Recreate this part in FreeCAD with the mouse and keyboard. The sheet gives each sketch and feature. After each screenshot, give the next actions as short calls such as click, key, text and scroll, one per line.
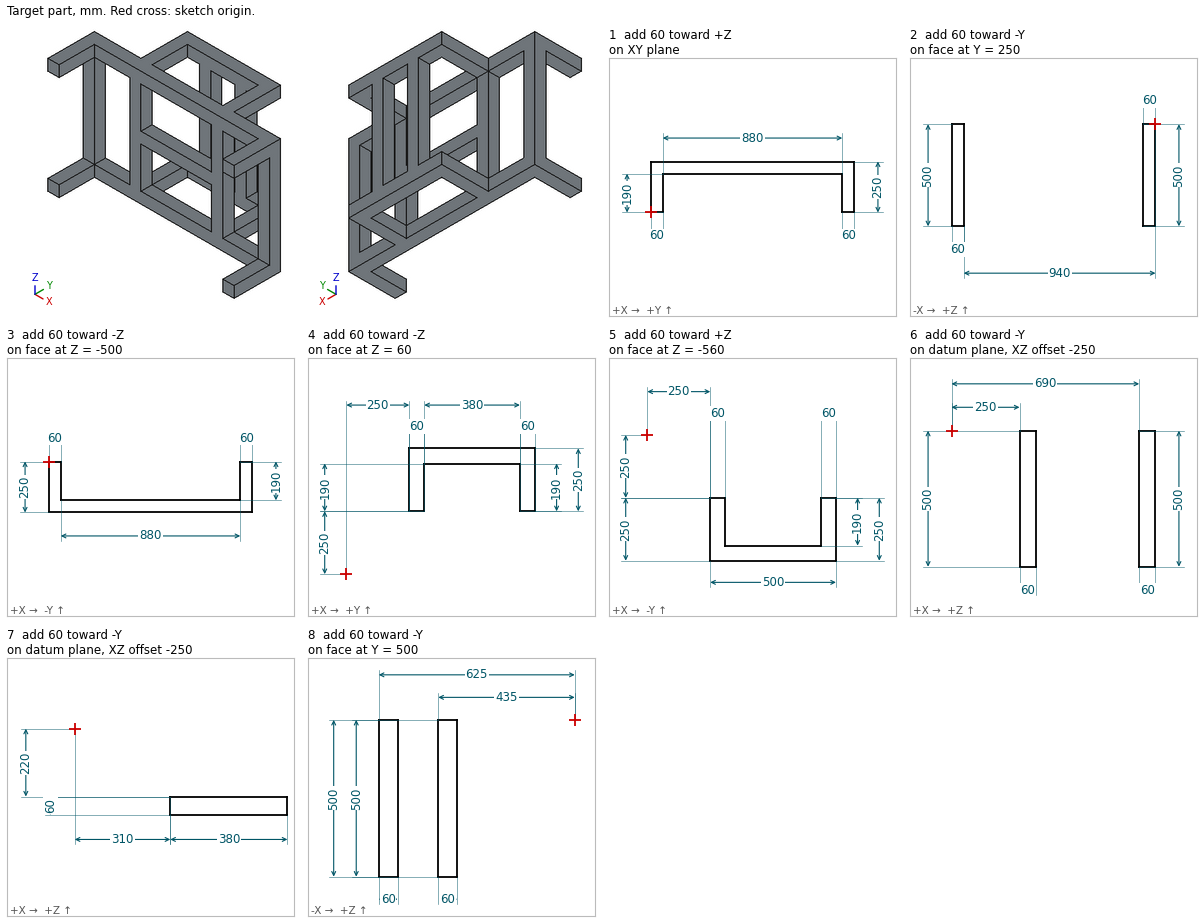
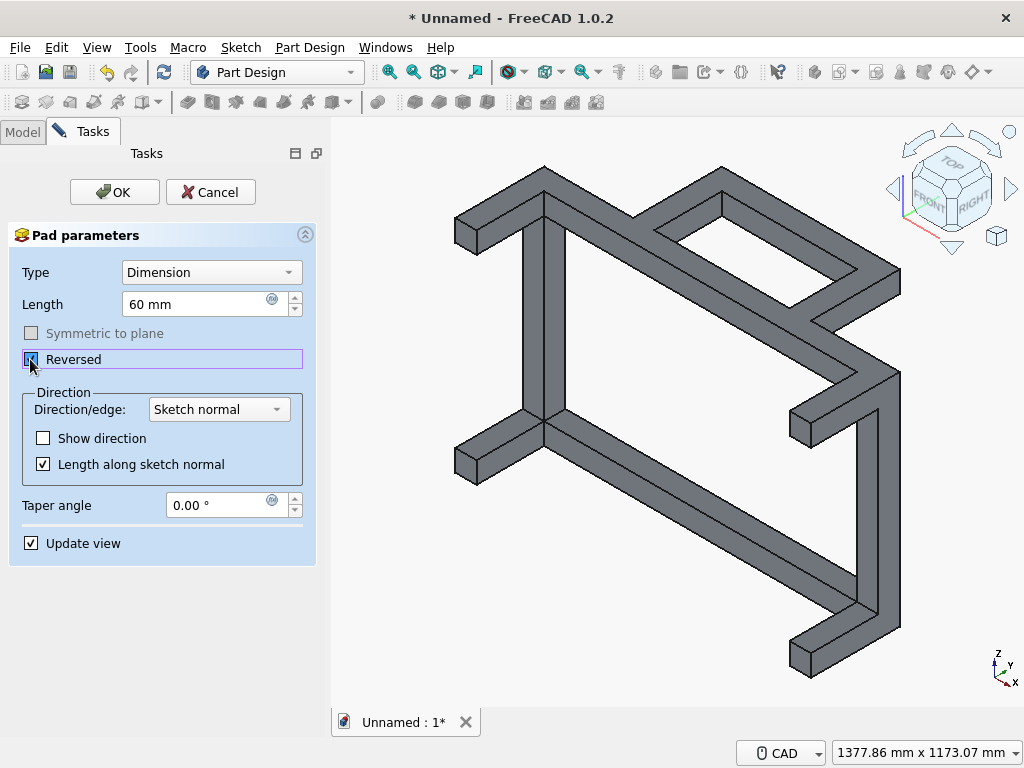
click(115, 192)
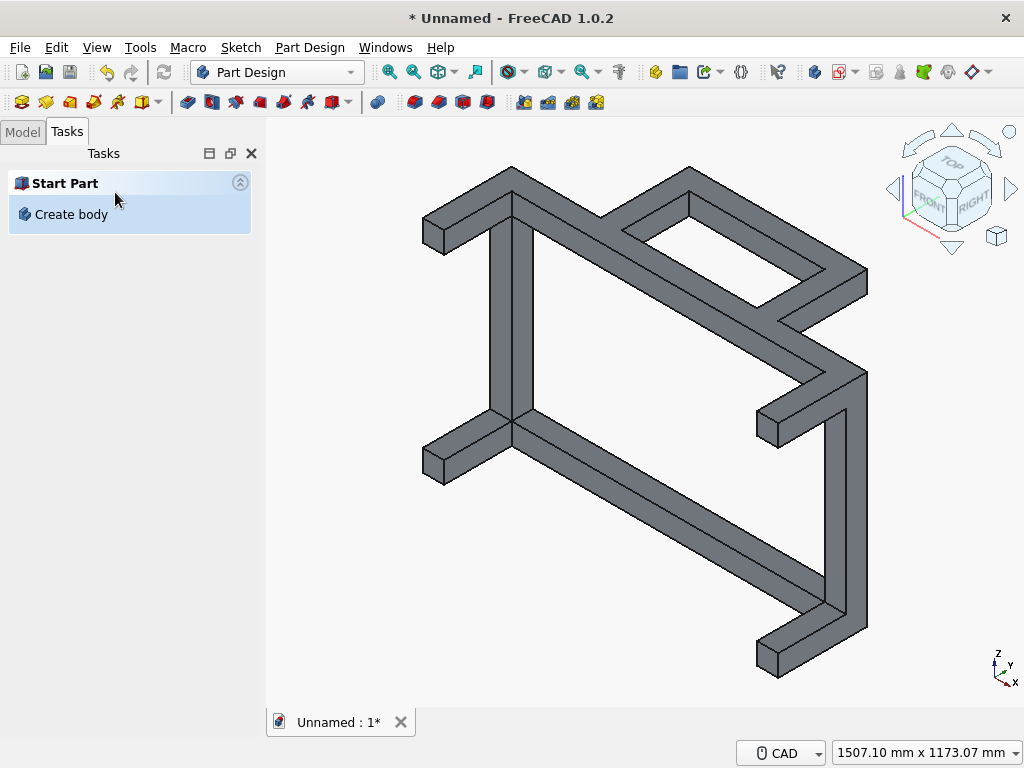
click(390, 72)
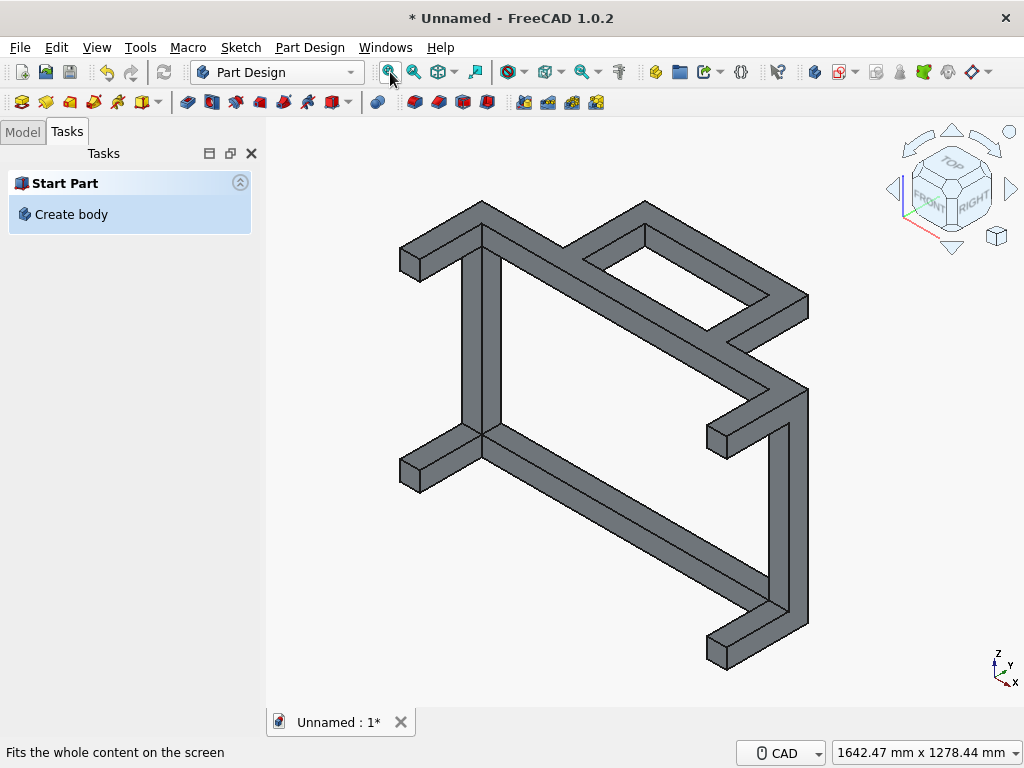
key(5)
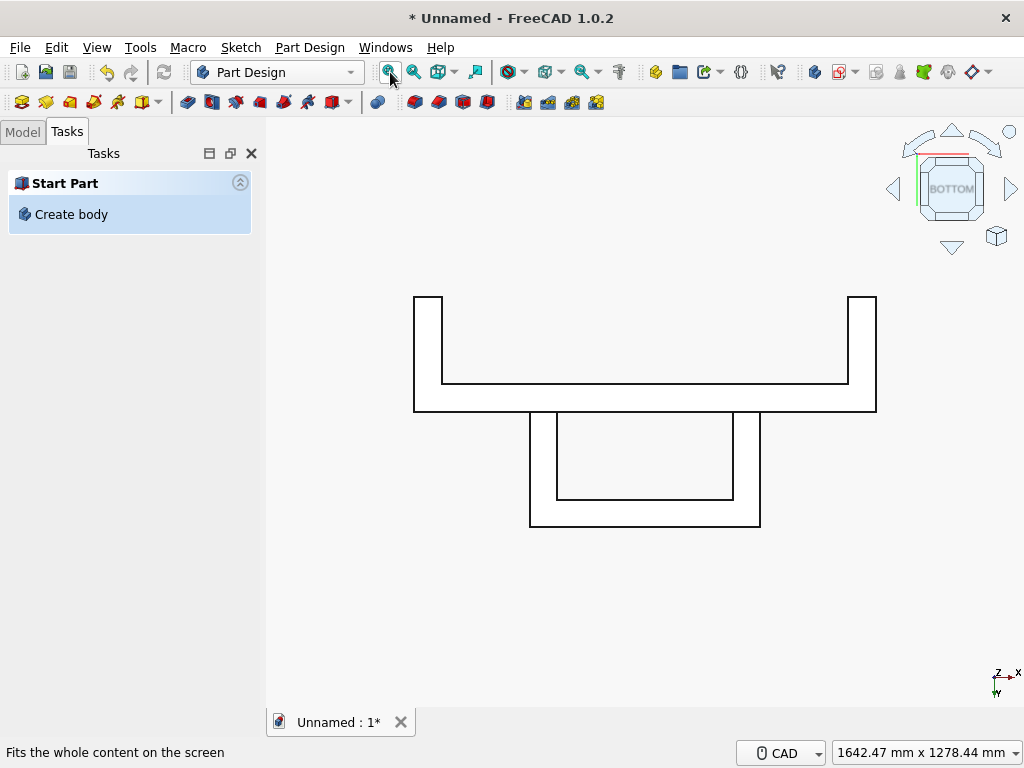
click(843, 403)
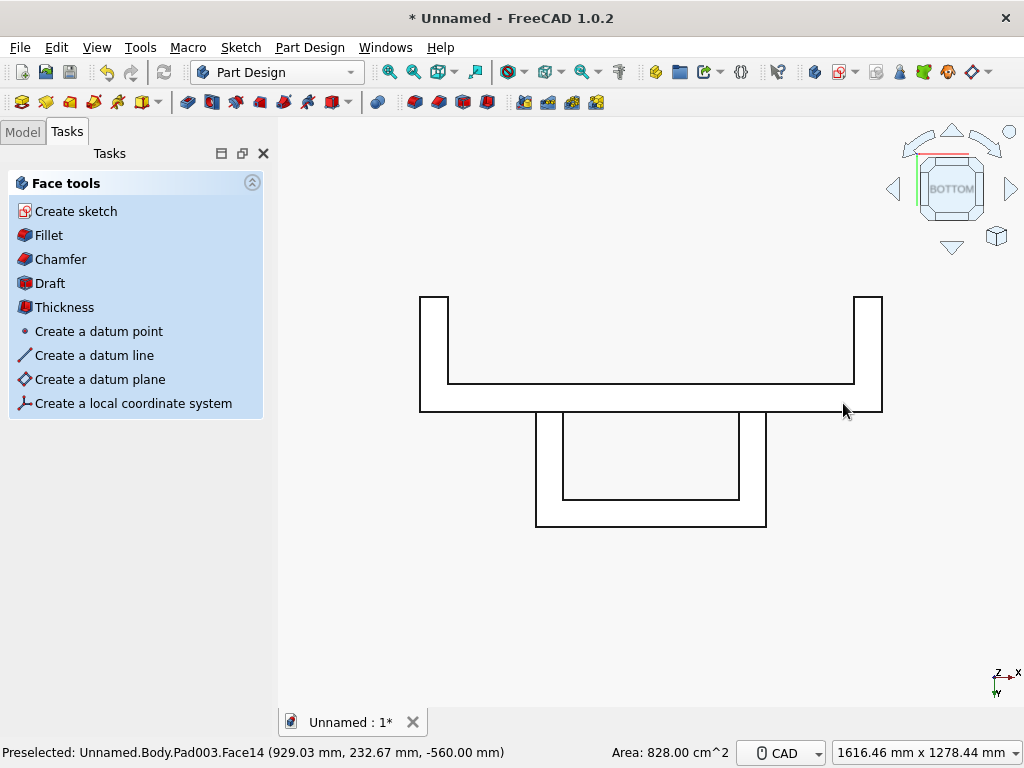
click(840, 72)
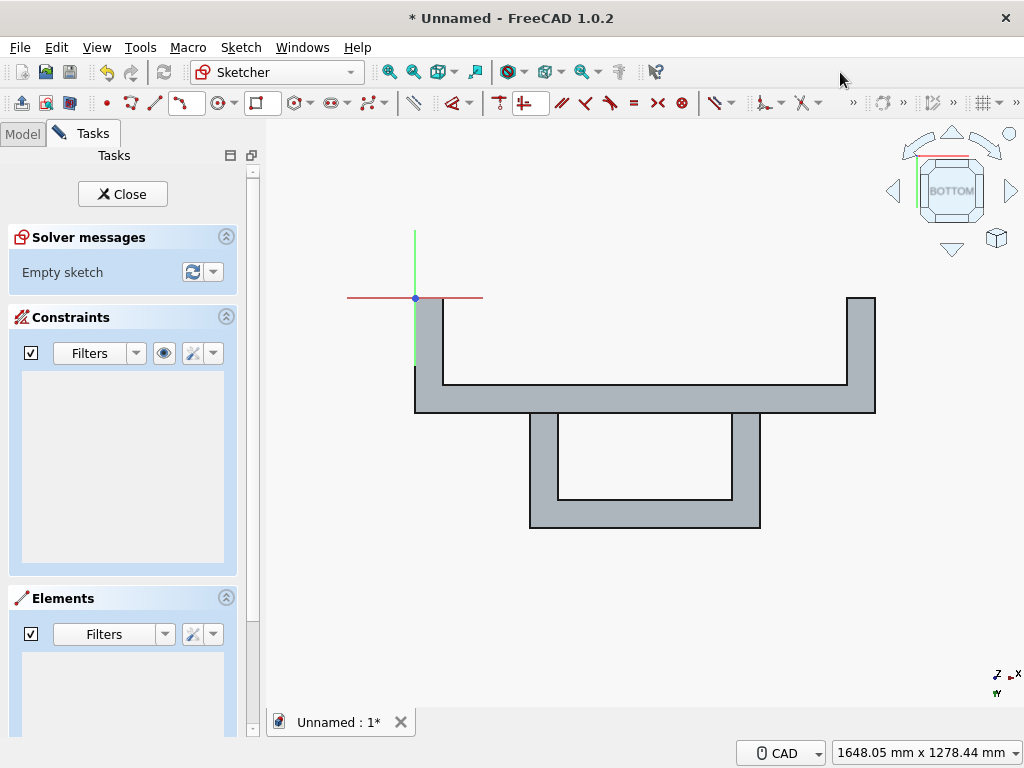
click(132, 104)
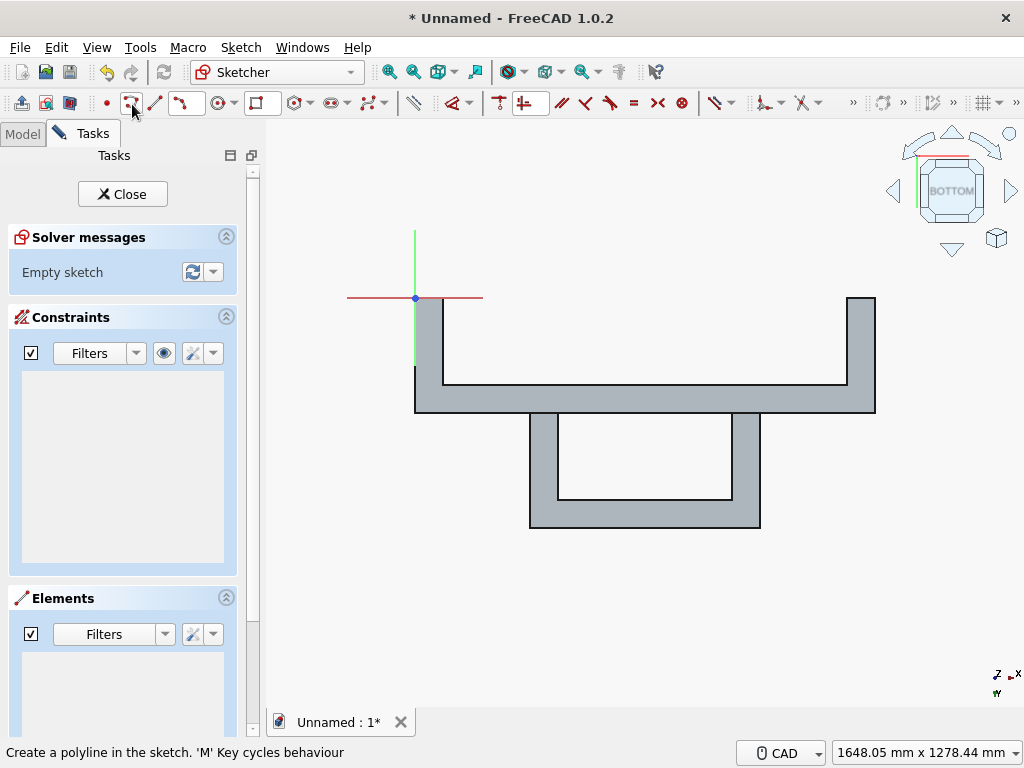
click(530, 413)
click(530, 528)
click(760, 528)
click(760, 413)
click(732, 413)
click(732, 500)
click(558, 500)
click(558, 413)
click(530, 414)
key(Escape)
key(Escape)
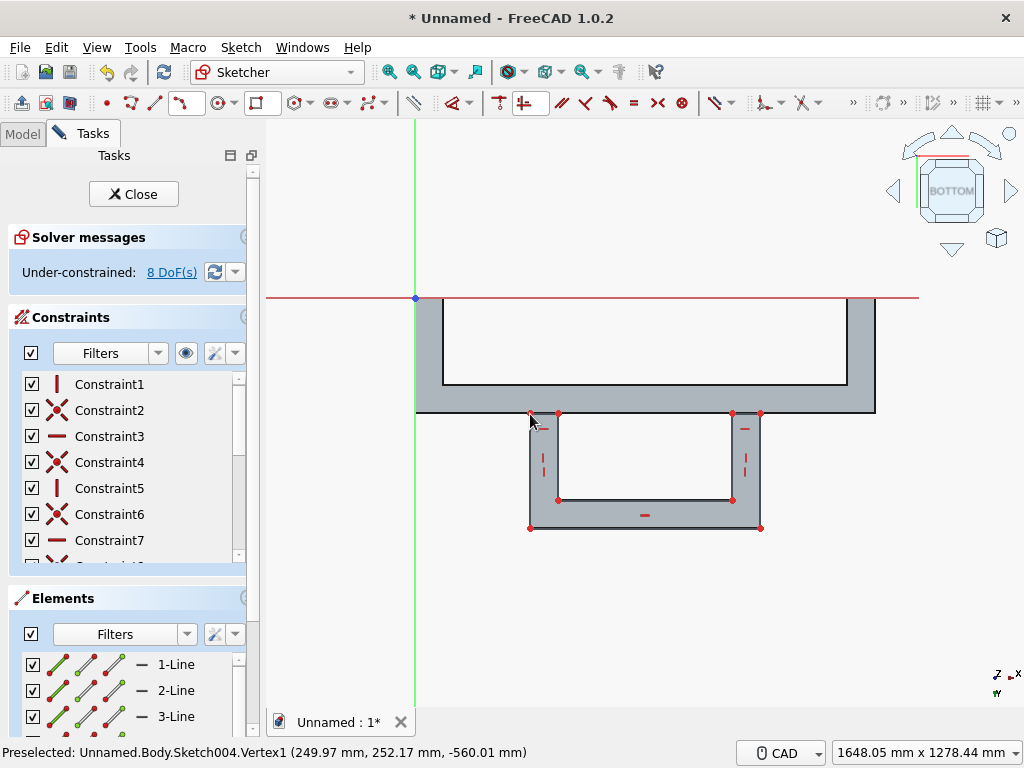
click(452, 104)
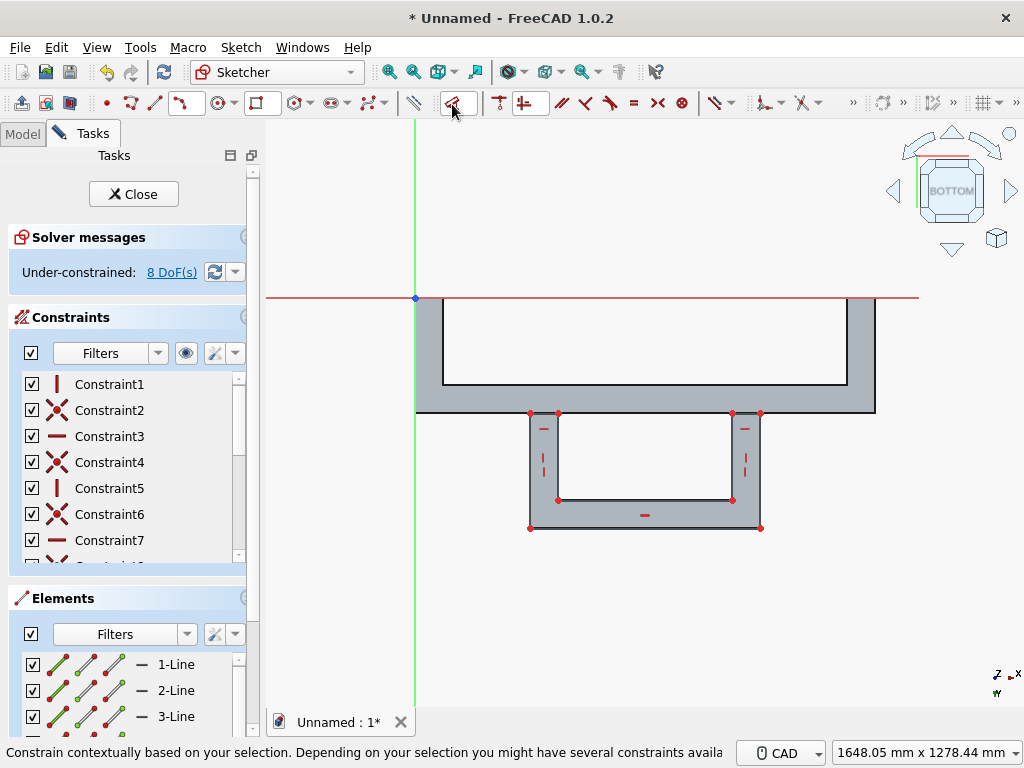
scroll(749, 414, up, 2)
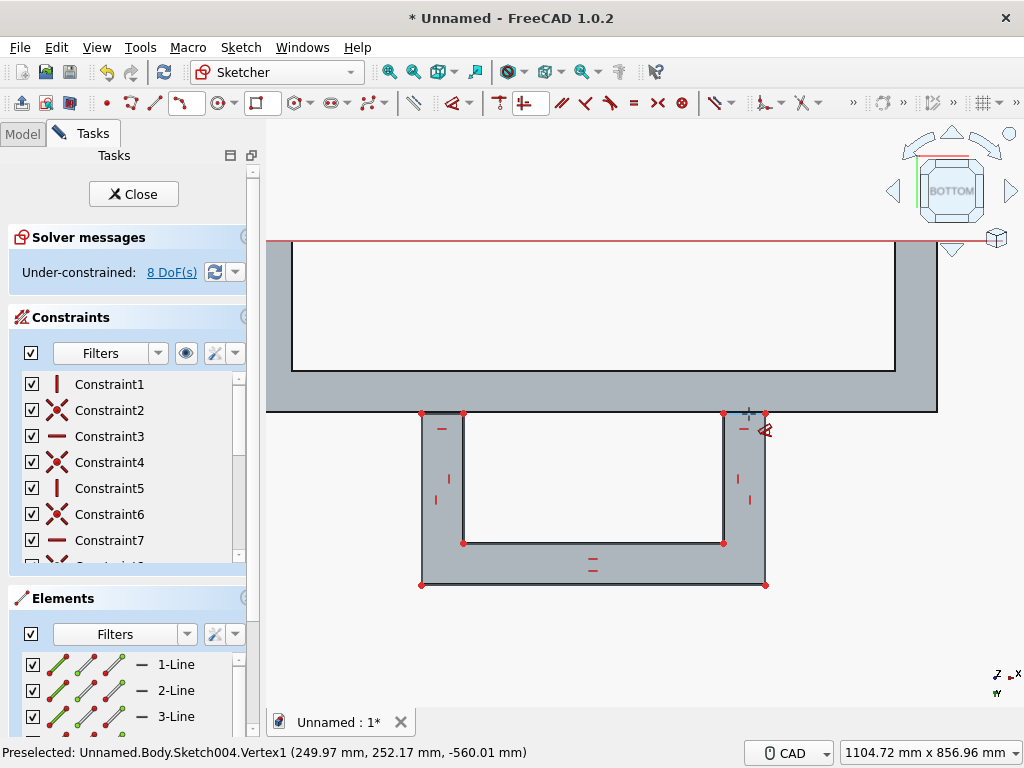
click(748, 414)
click(744, 448)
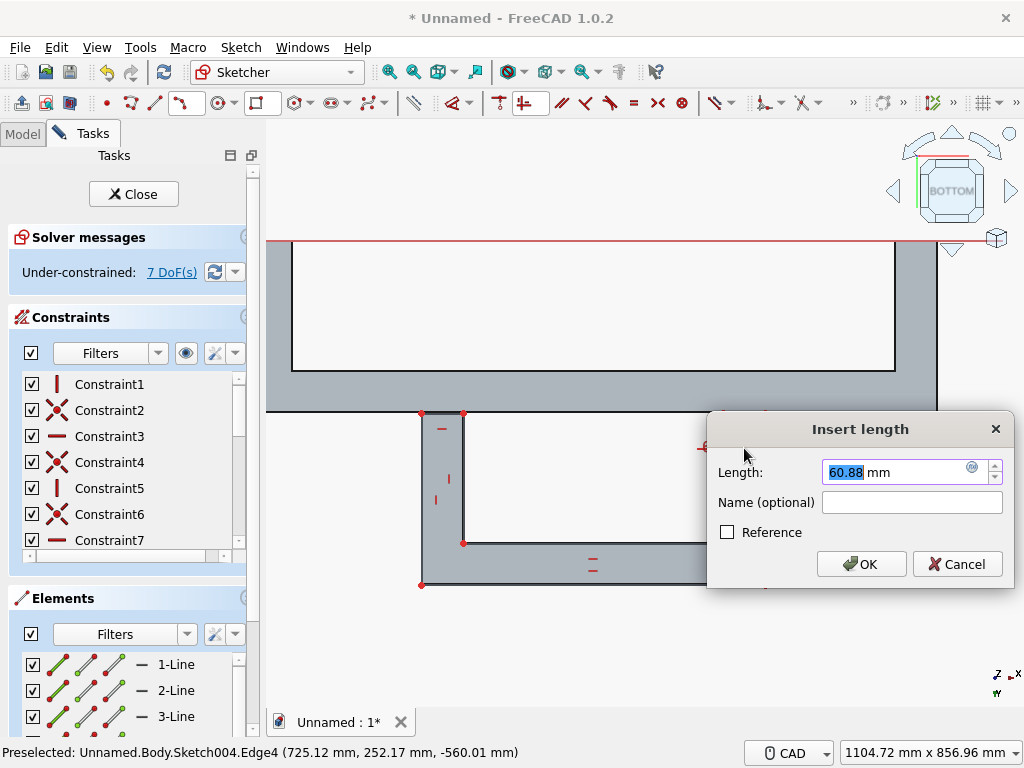
text(60)
key(Return)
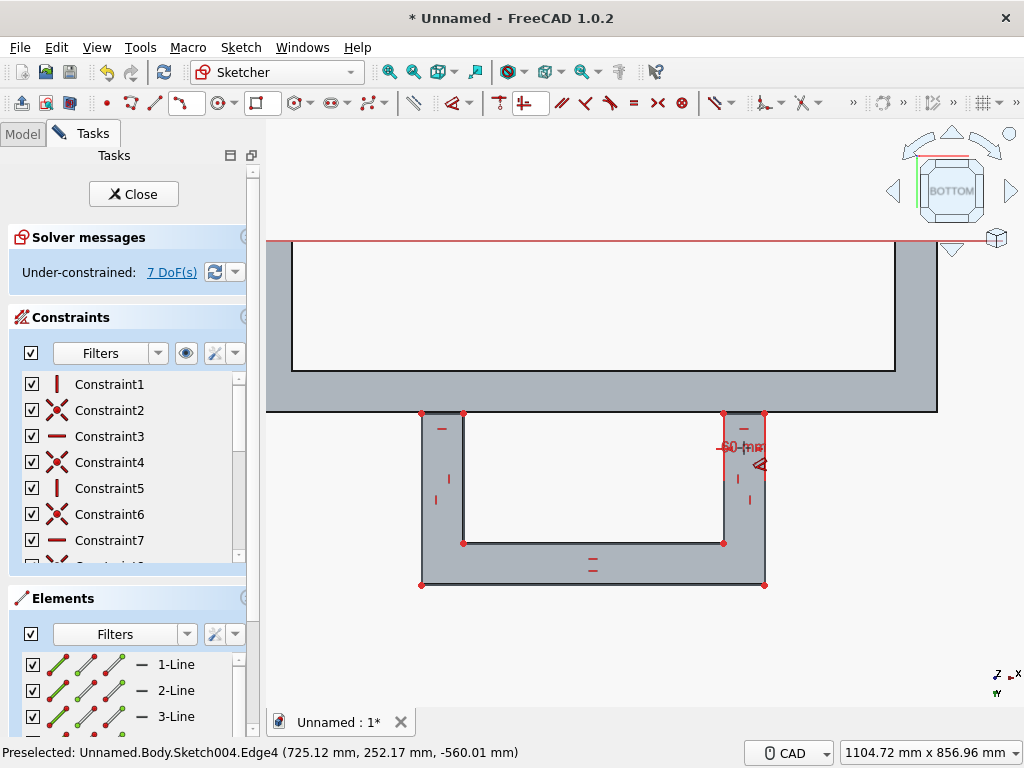
click(451, 414)
click(443, 448)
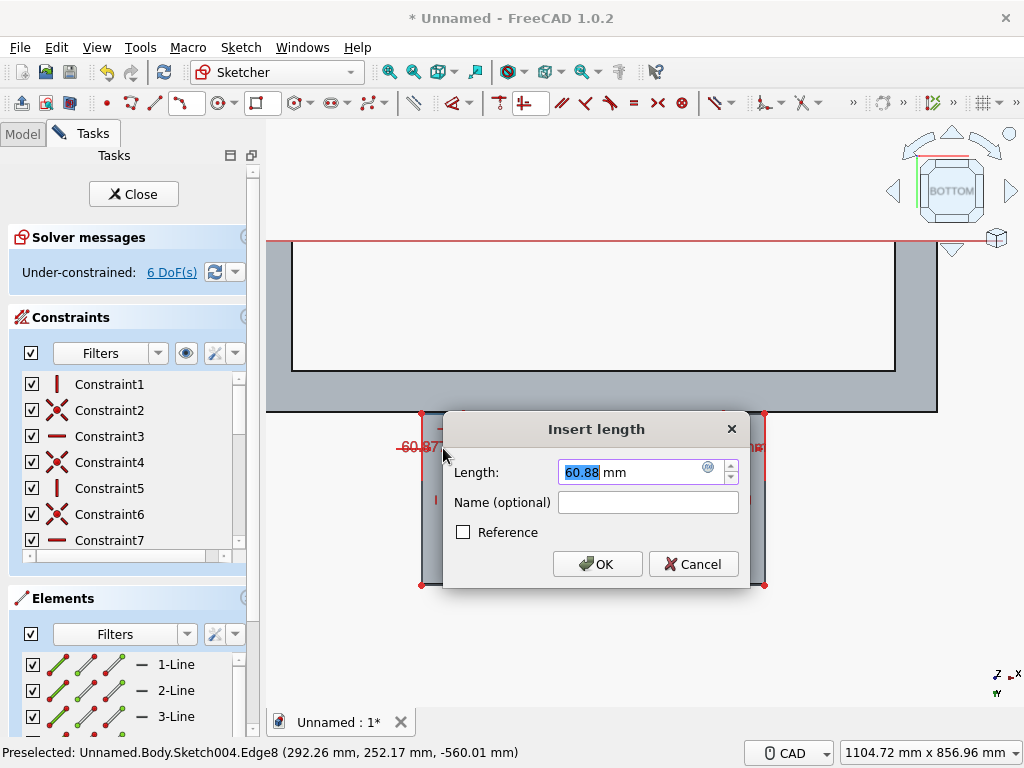
text(60)
key(Return)